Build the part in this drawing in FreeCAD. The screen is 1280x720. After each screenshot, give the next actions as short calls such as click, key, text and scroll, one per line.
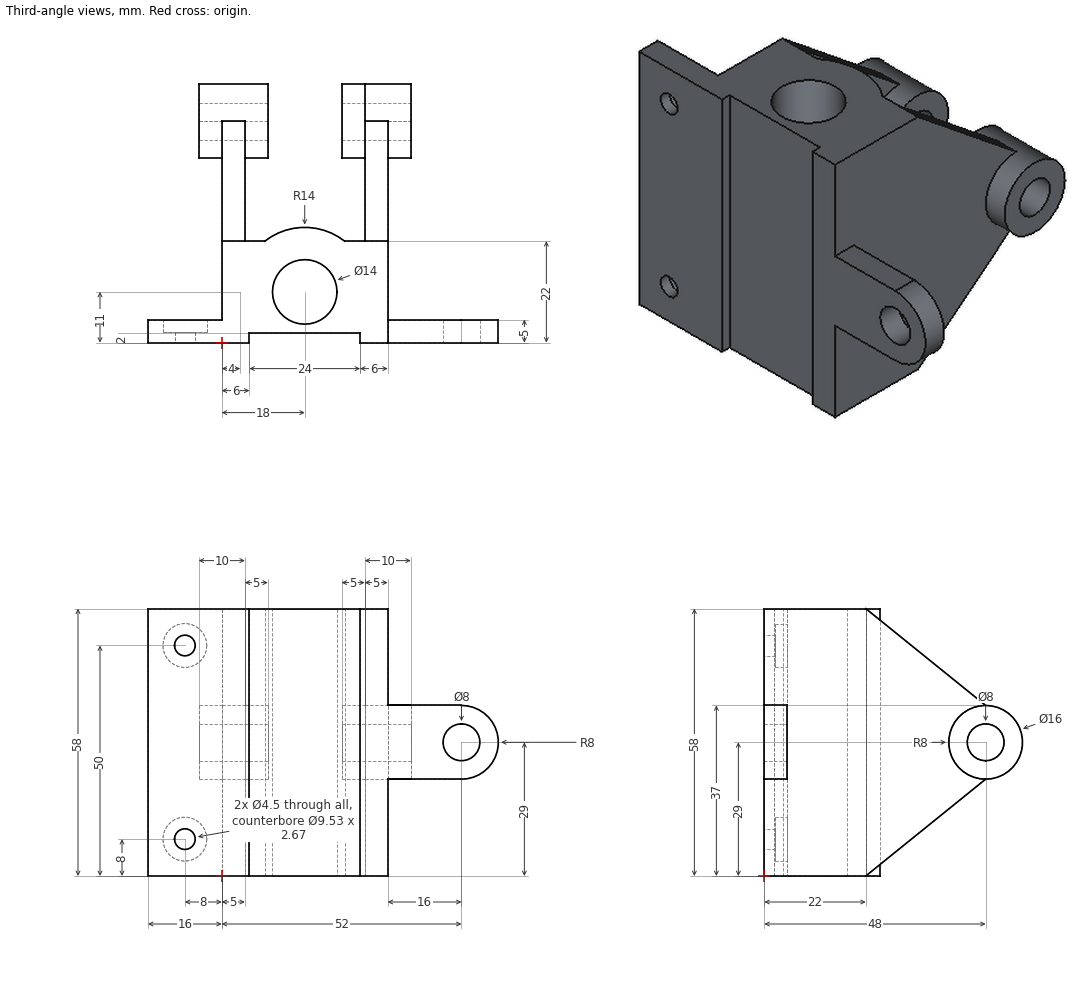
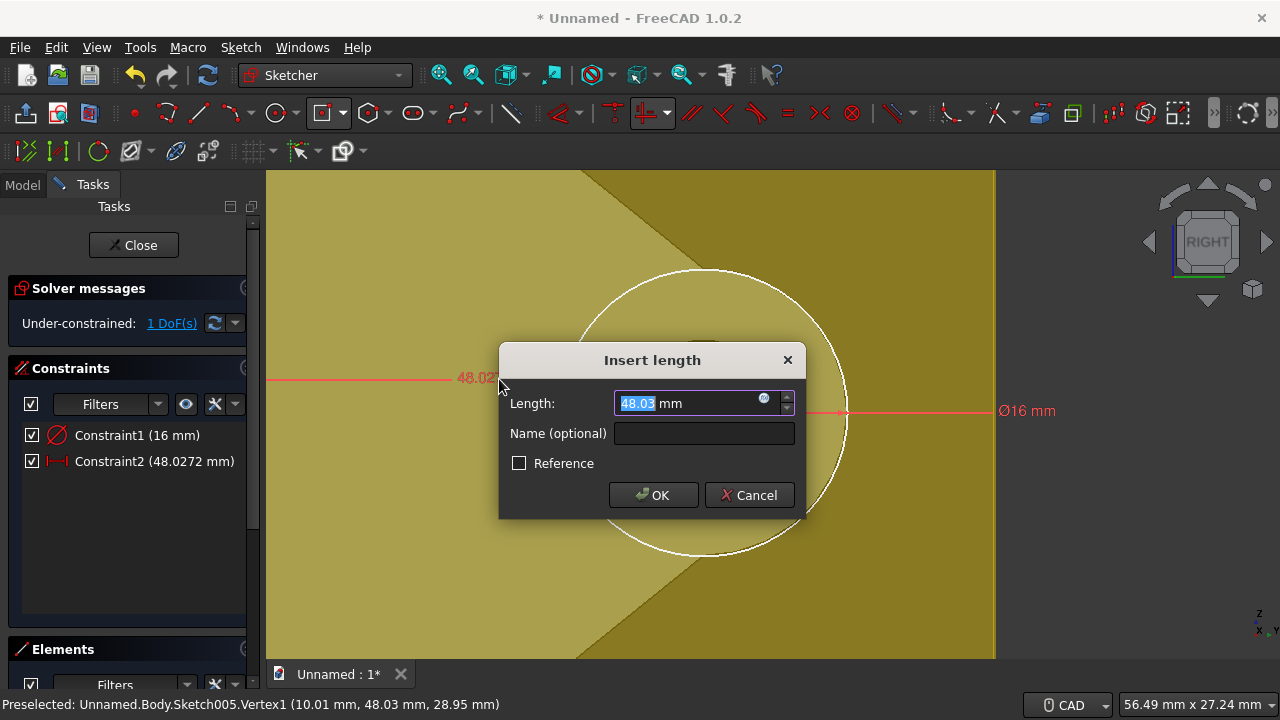
text(48)
key(Return)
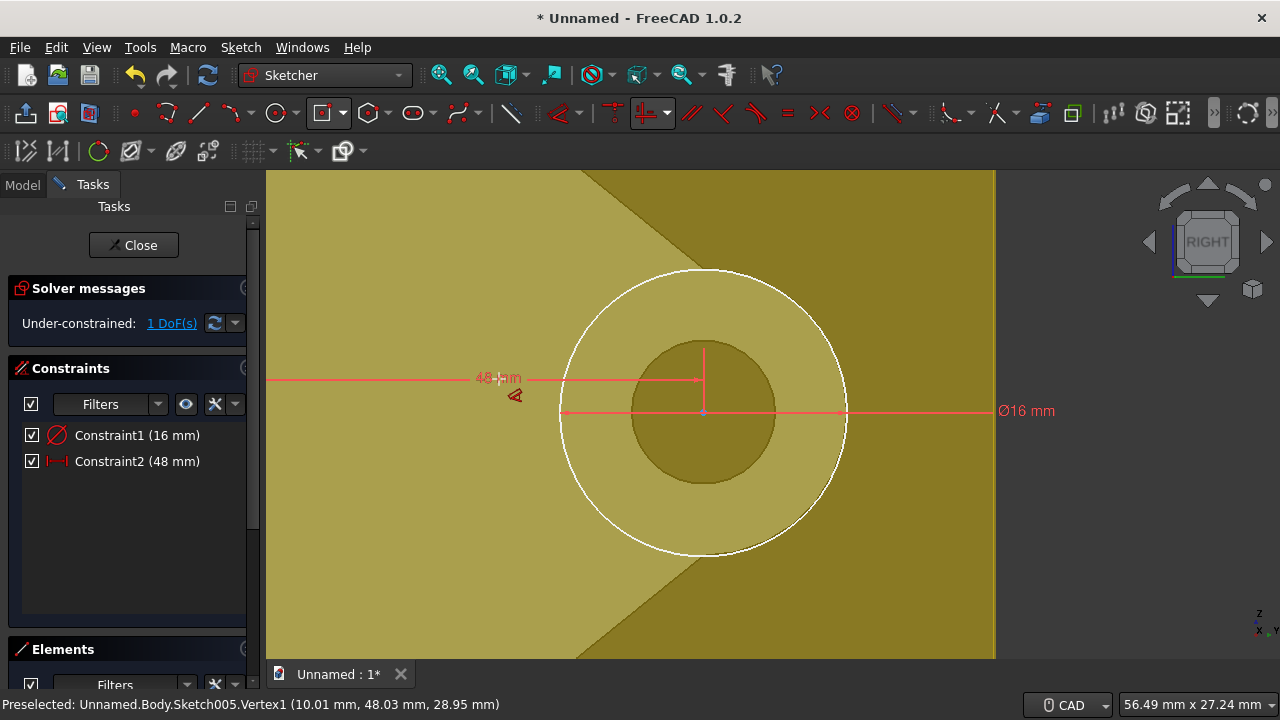
click(704, 413)
click(738, 522)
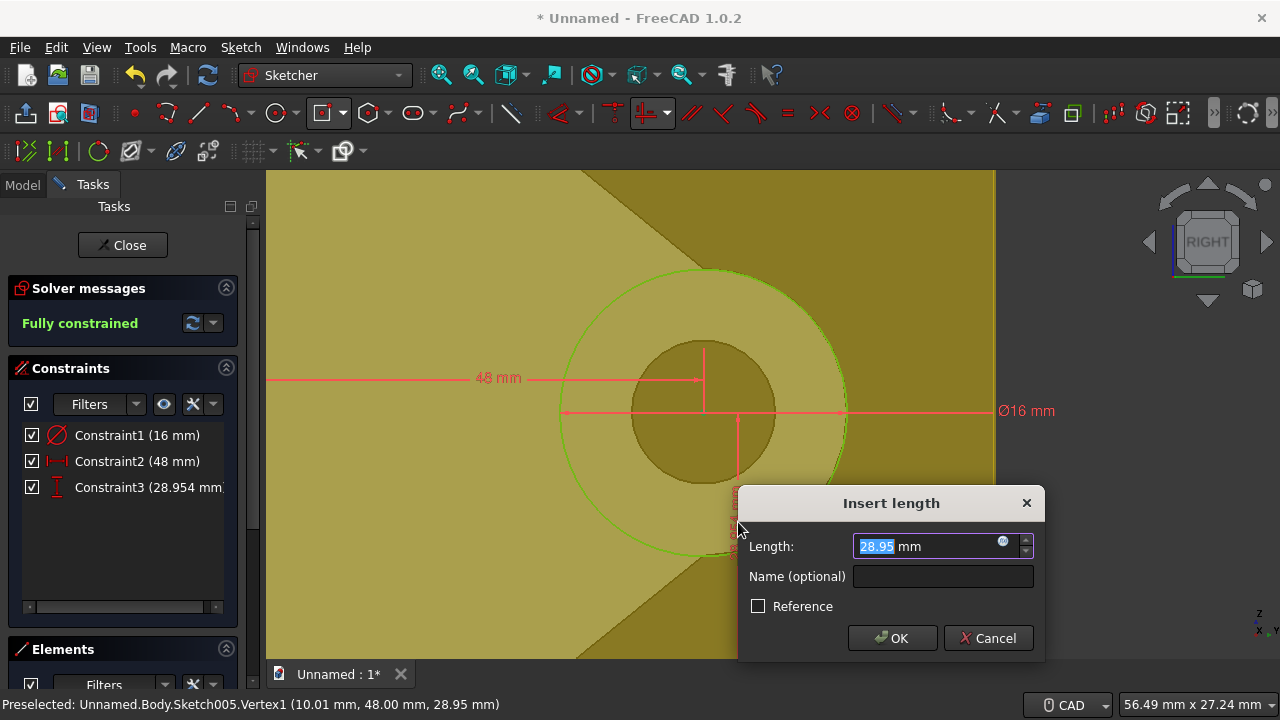
text(29)
key(Return)
key(Escape)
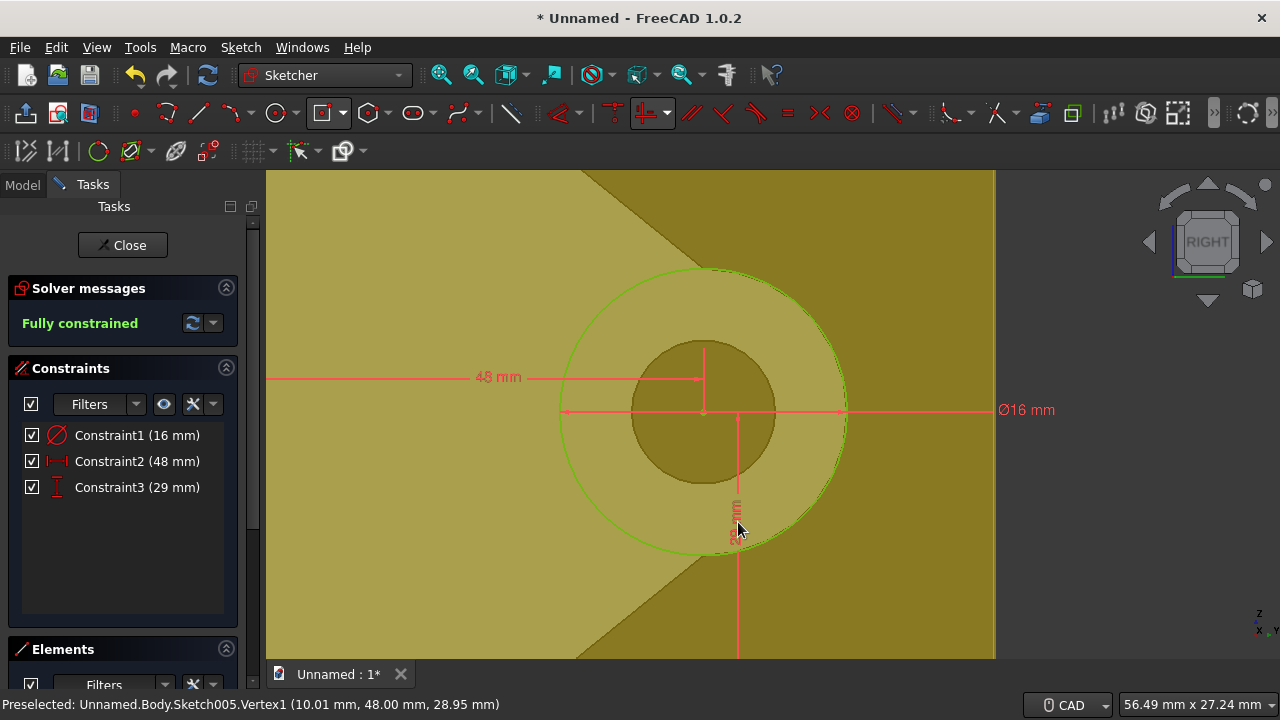
click(123, 245)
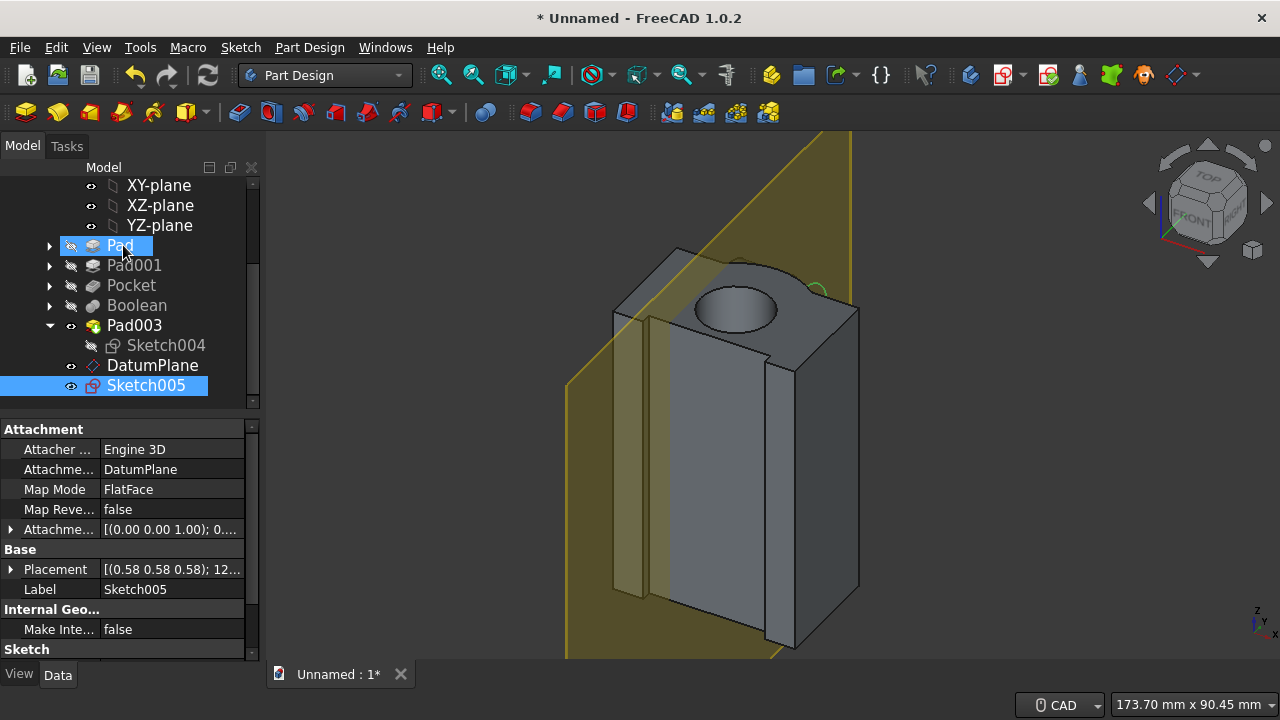
click(26, 112)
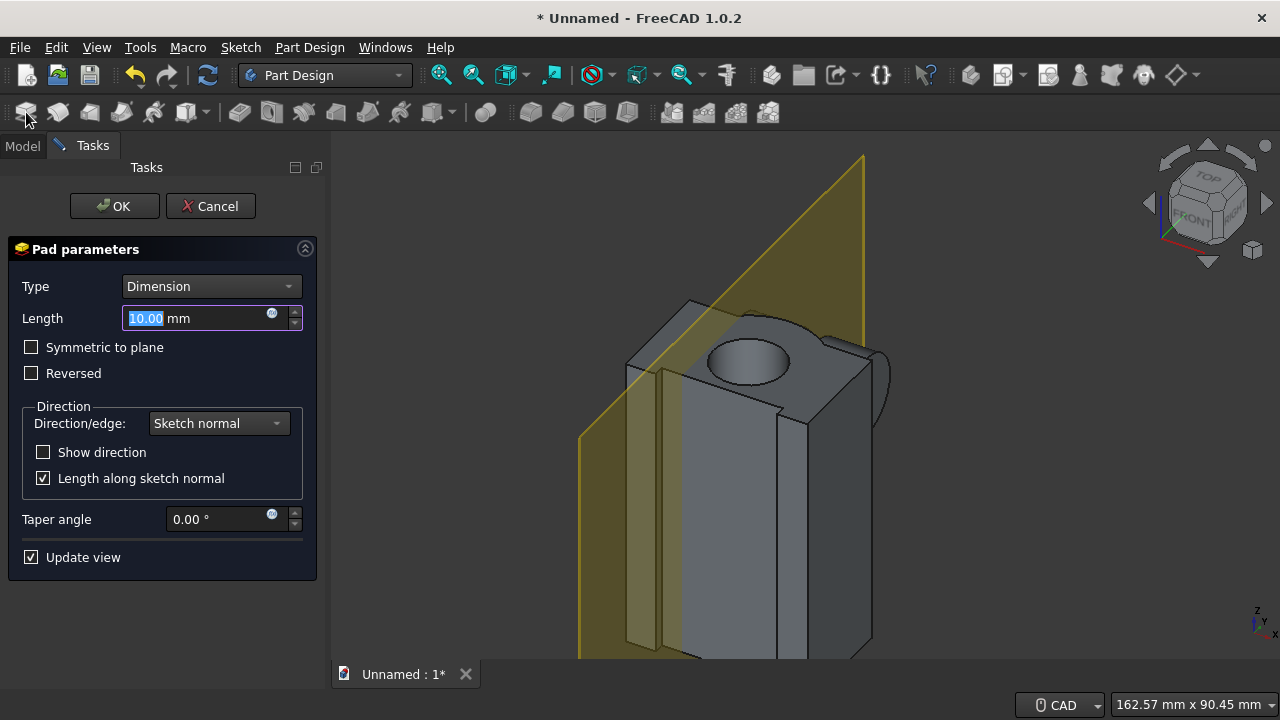
text(5)
key(Tab)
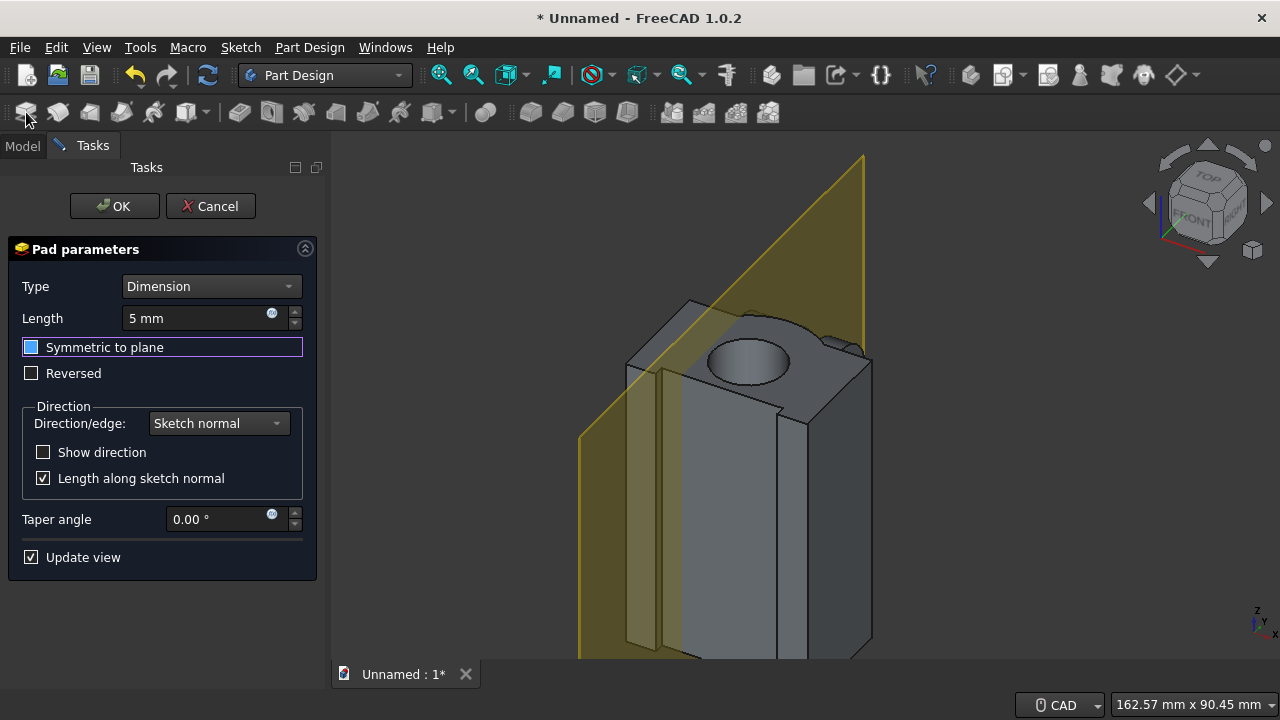
click(30, 373)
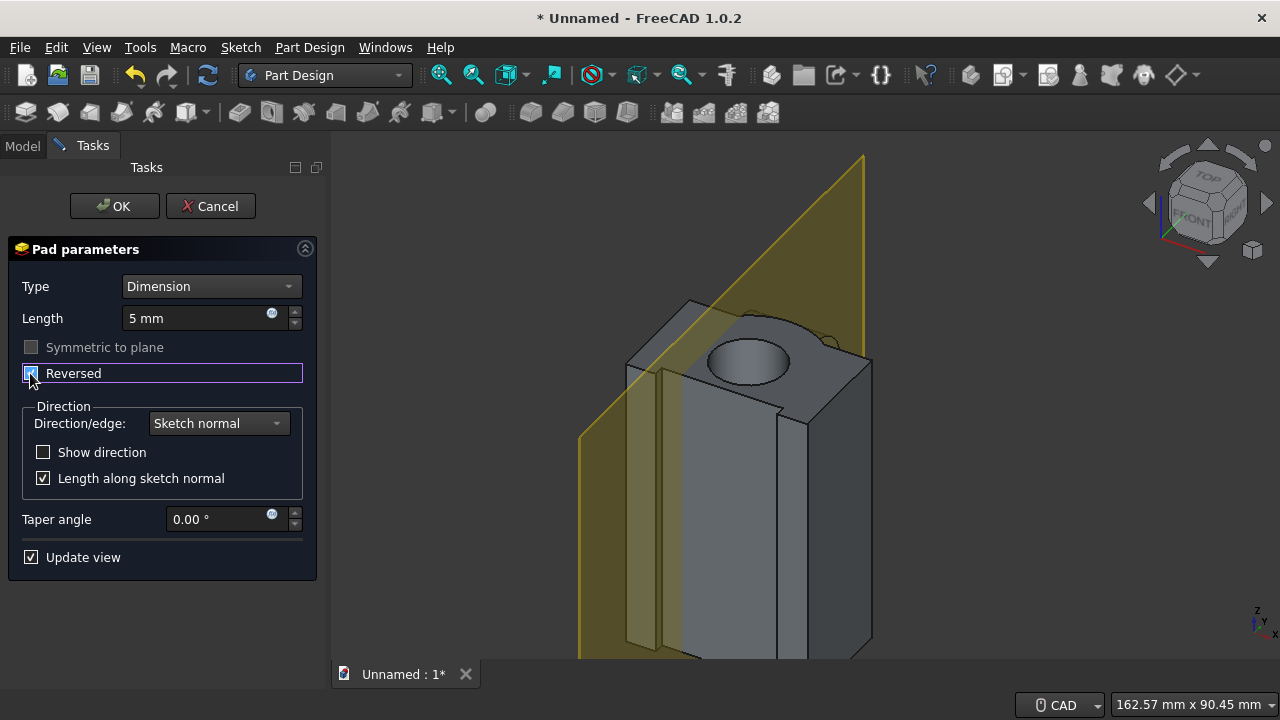
click(115, 206)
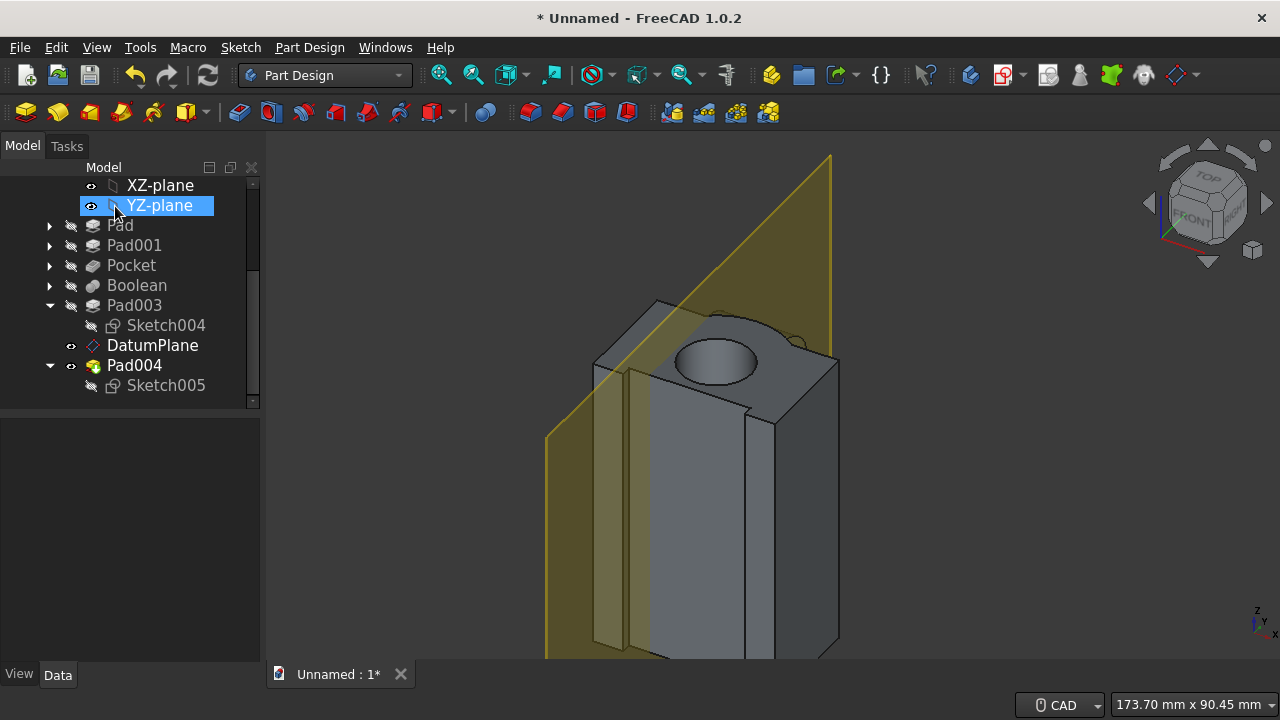
click(116, 346)
key(space)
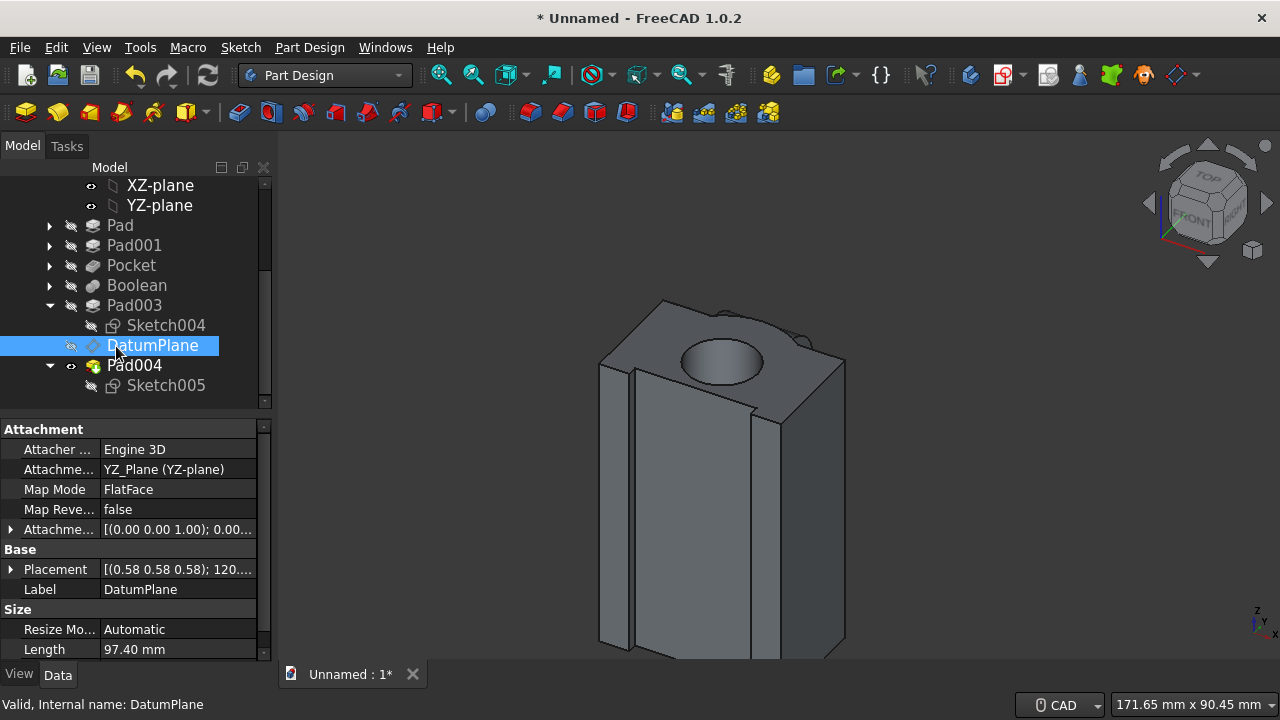
key(v)
key(f)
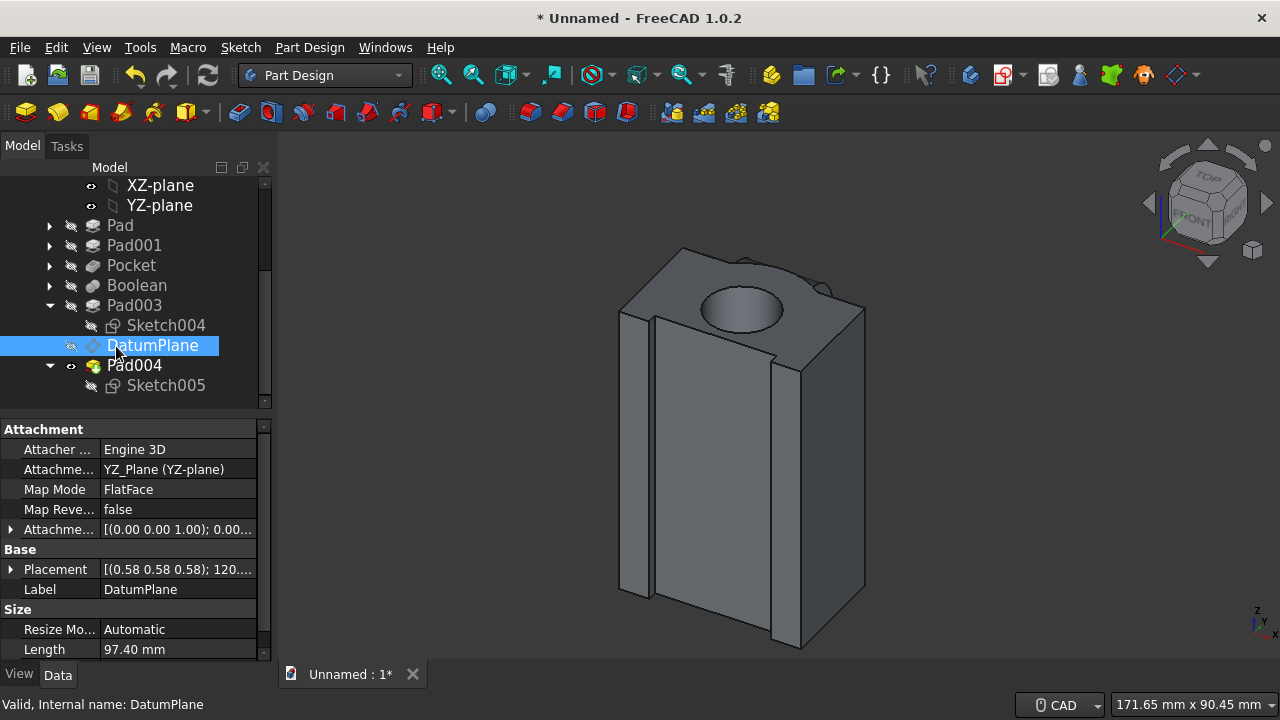
key(0)